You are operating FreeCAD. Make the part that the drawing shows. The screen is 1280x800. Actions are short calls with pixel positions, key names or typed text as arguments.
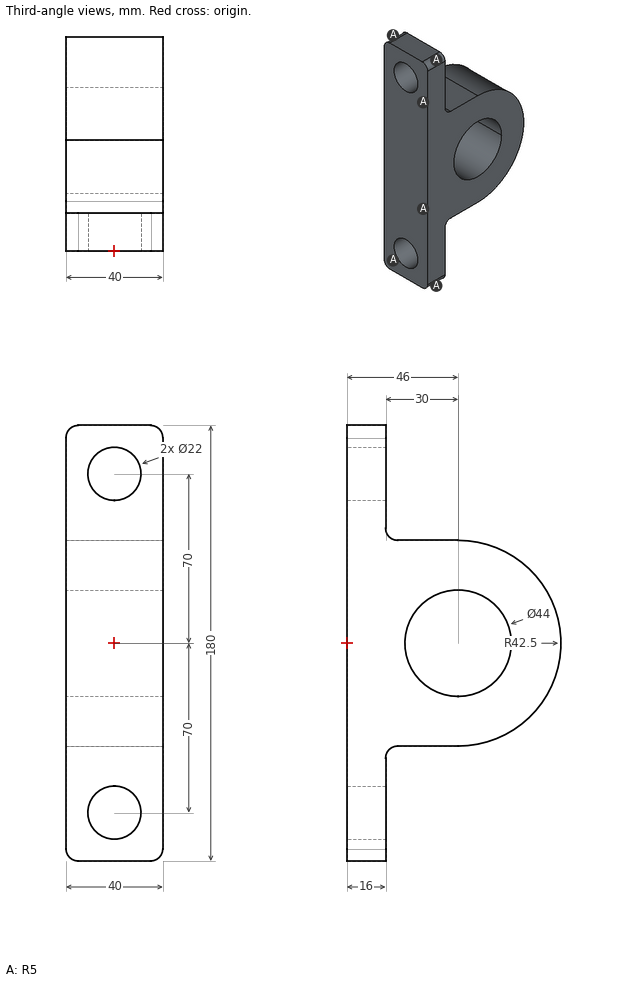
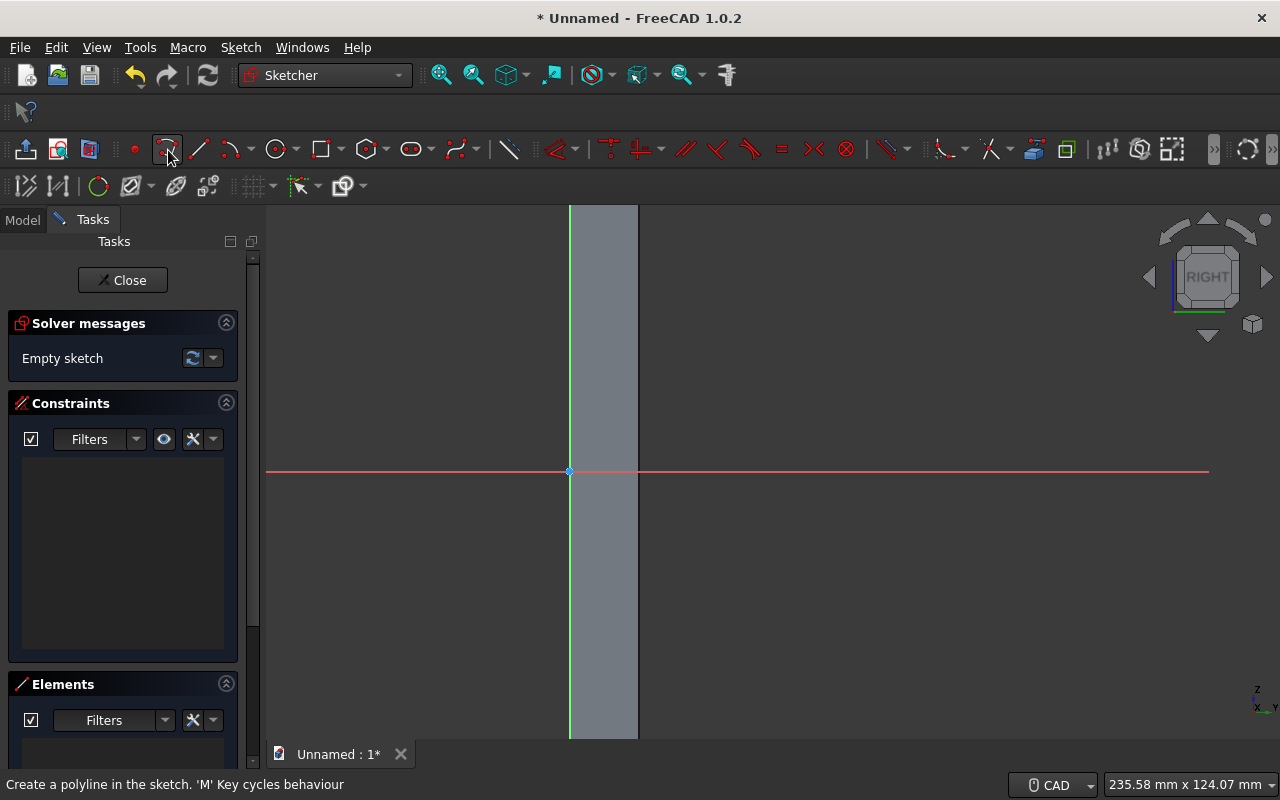
click(768, 289)
click(639, 289)
click(639, 655)
click(768, 655)
right_click(768, 655)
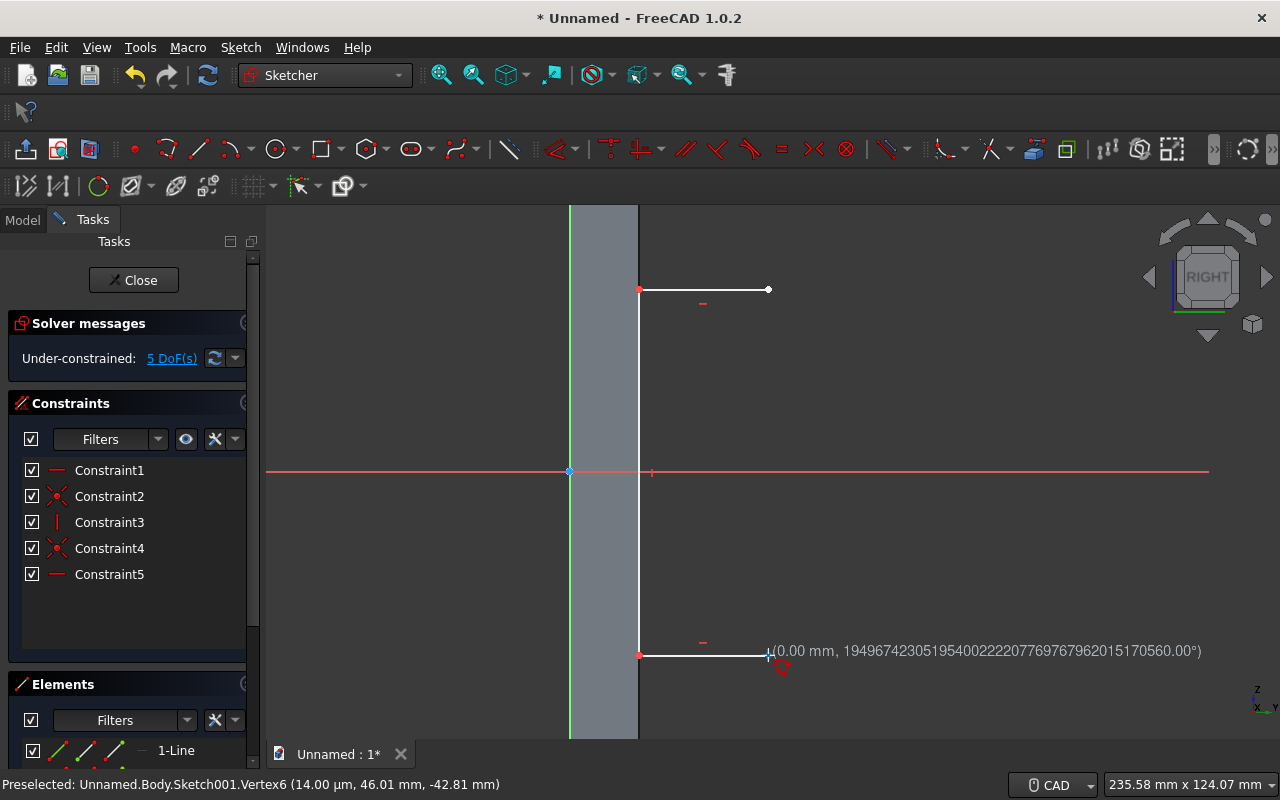
click(254, 150)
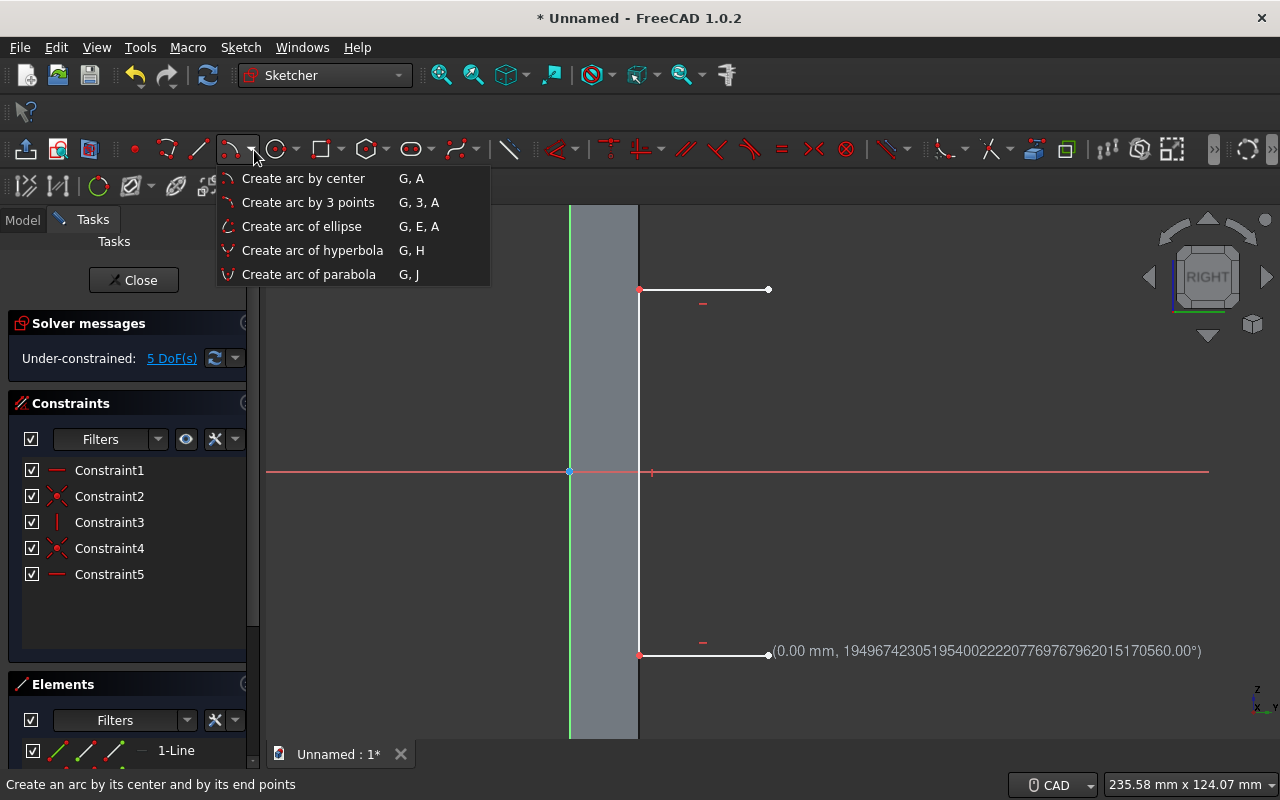
click(354, 202)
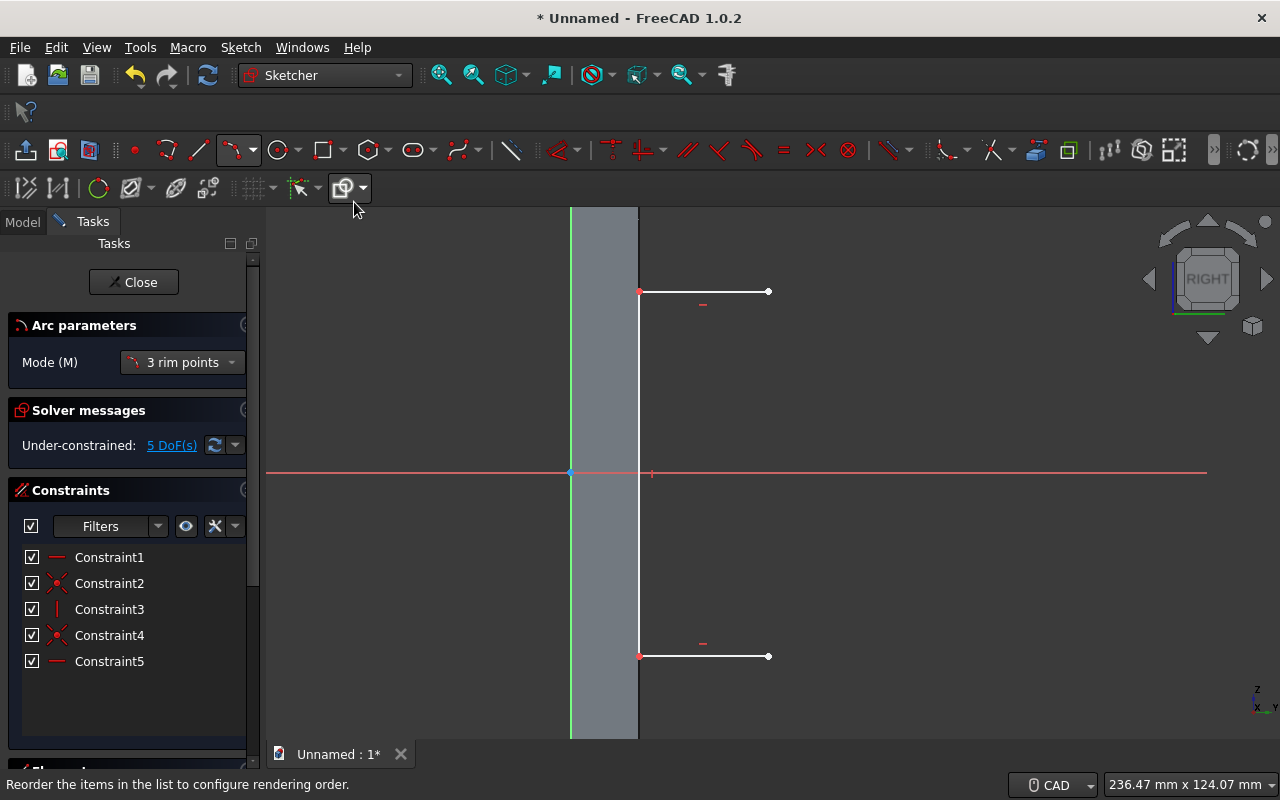
click(768, 656)
click(768, 292)
click(941, 529)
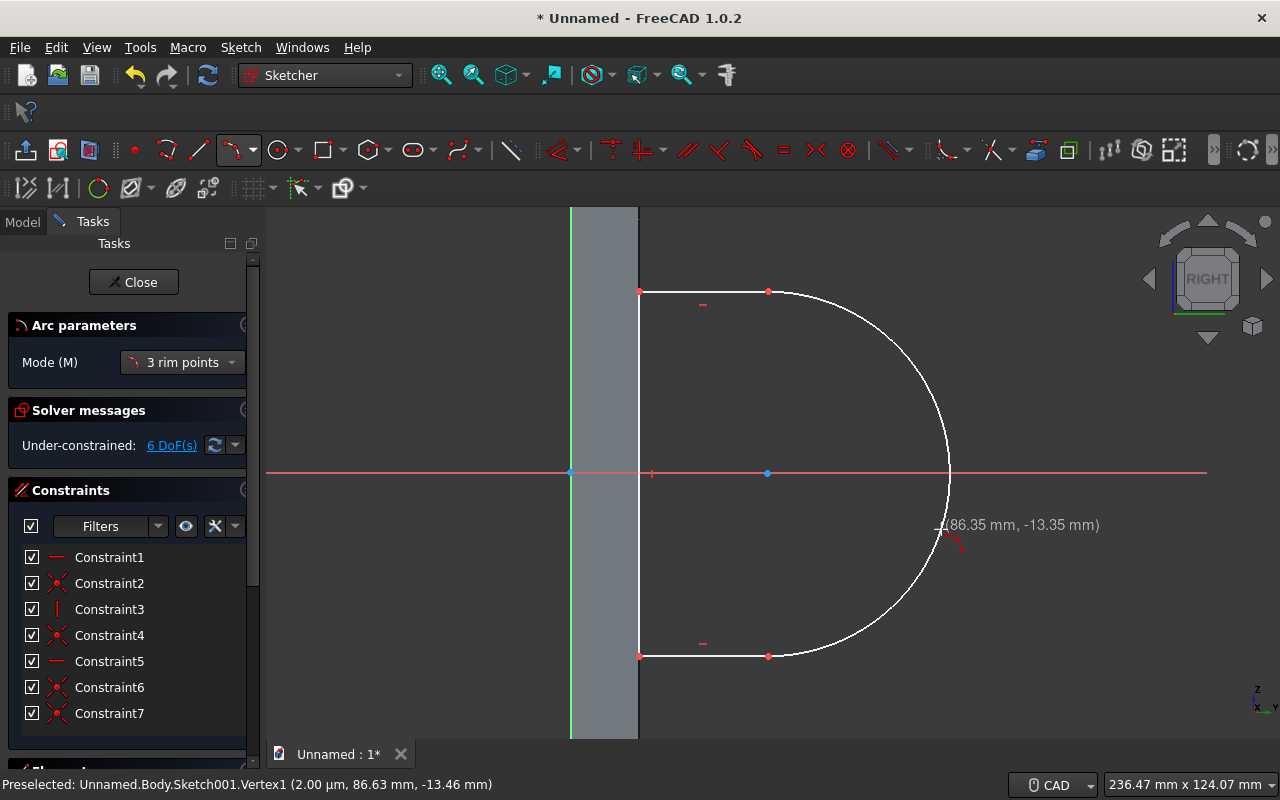
key(g)
key(c)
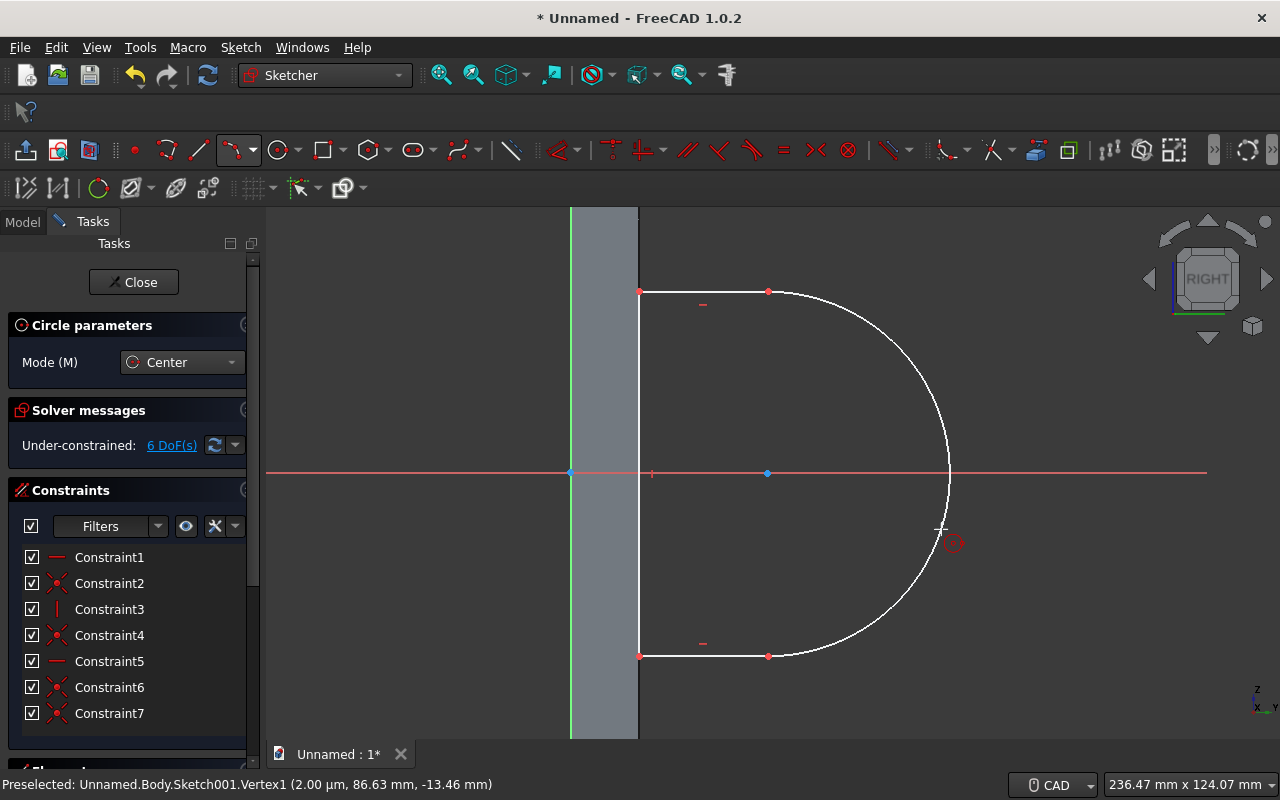
click(768, 473)
click(835, 406)
key(Escape)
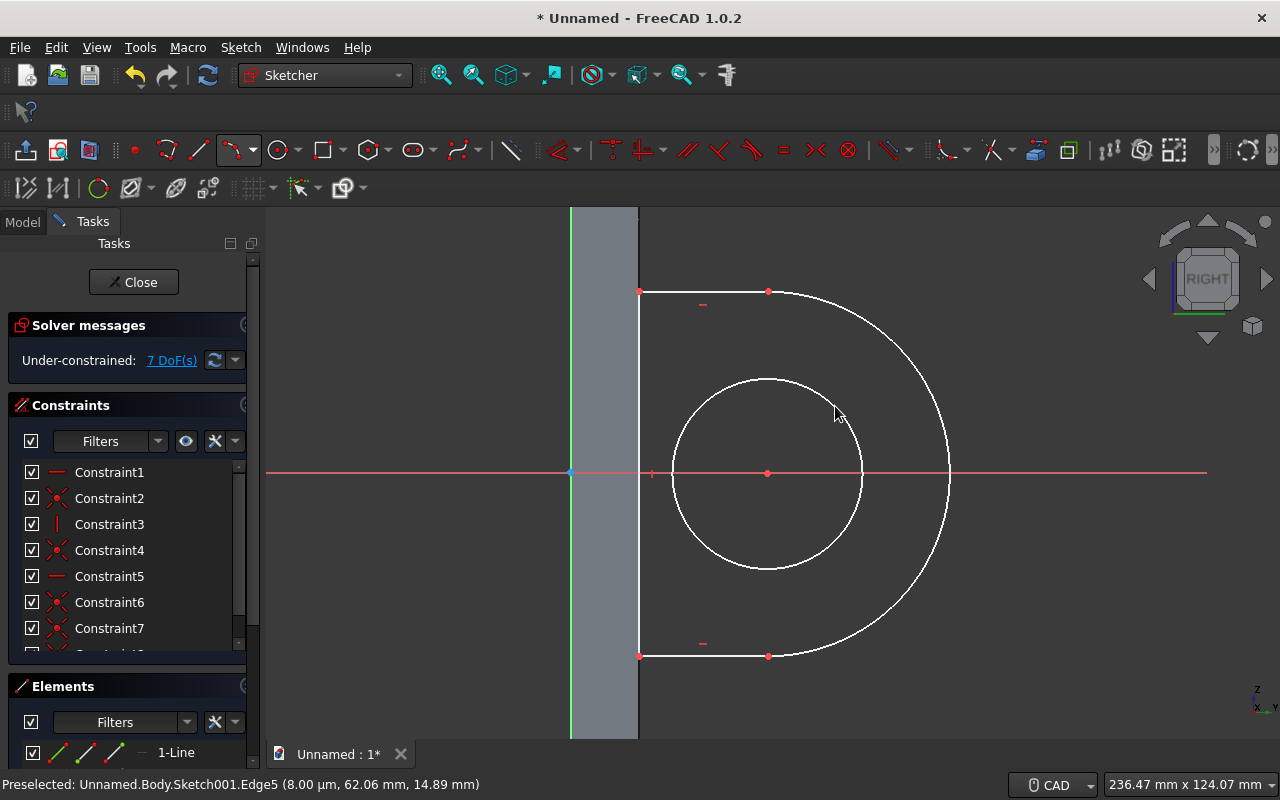
click(767, 474)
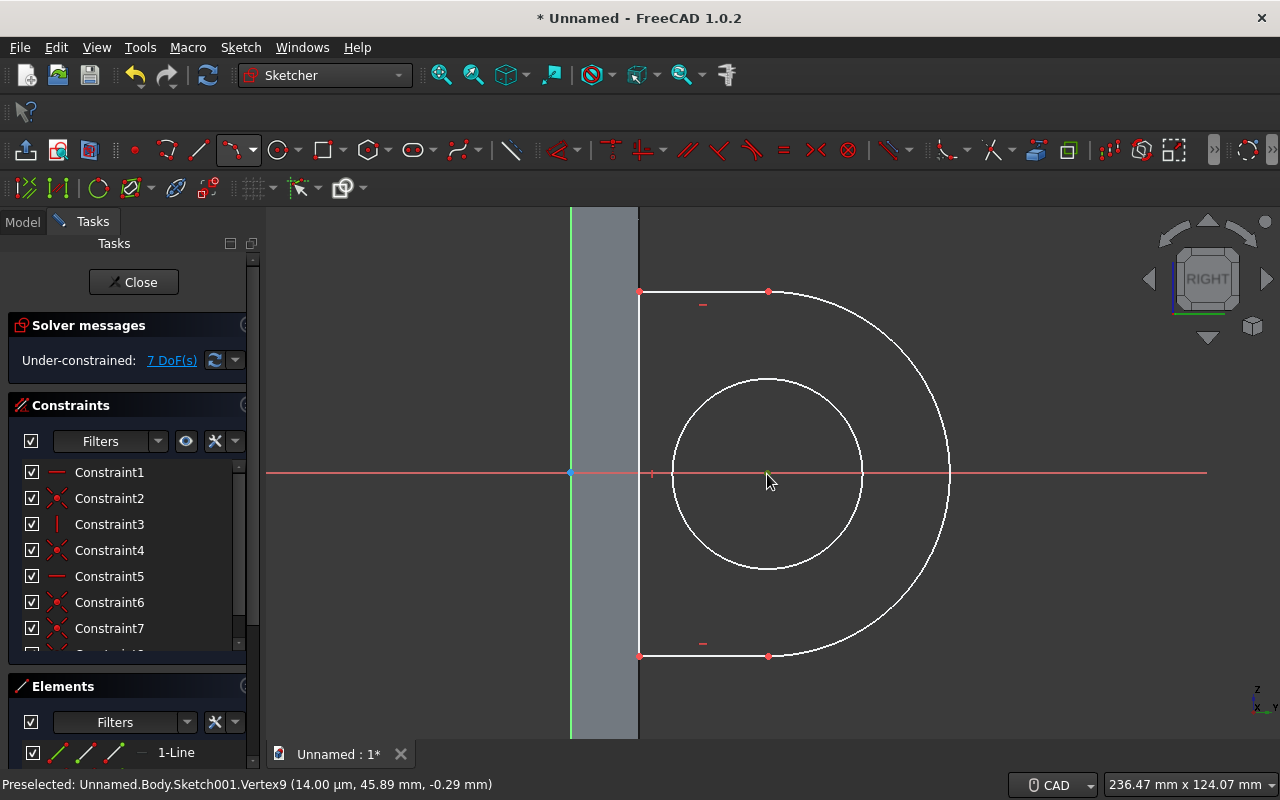
click(353, 473)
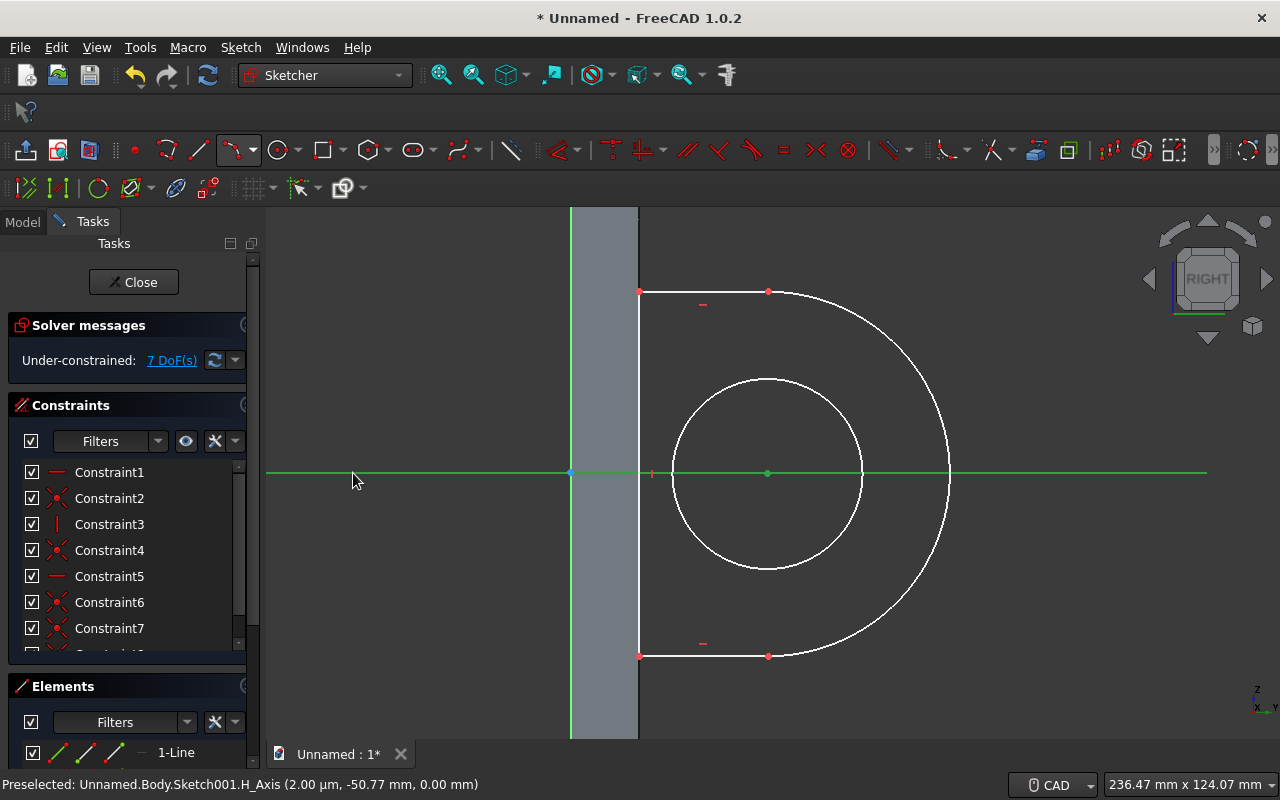
click(612, 150)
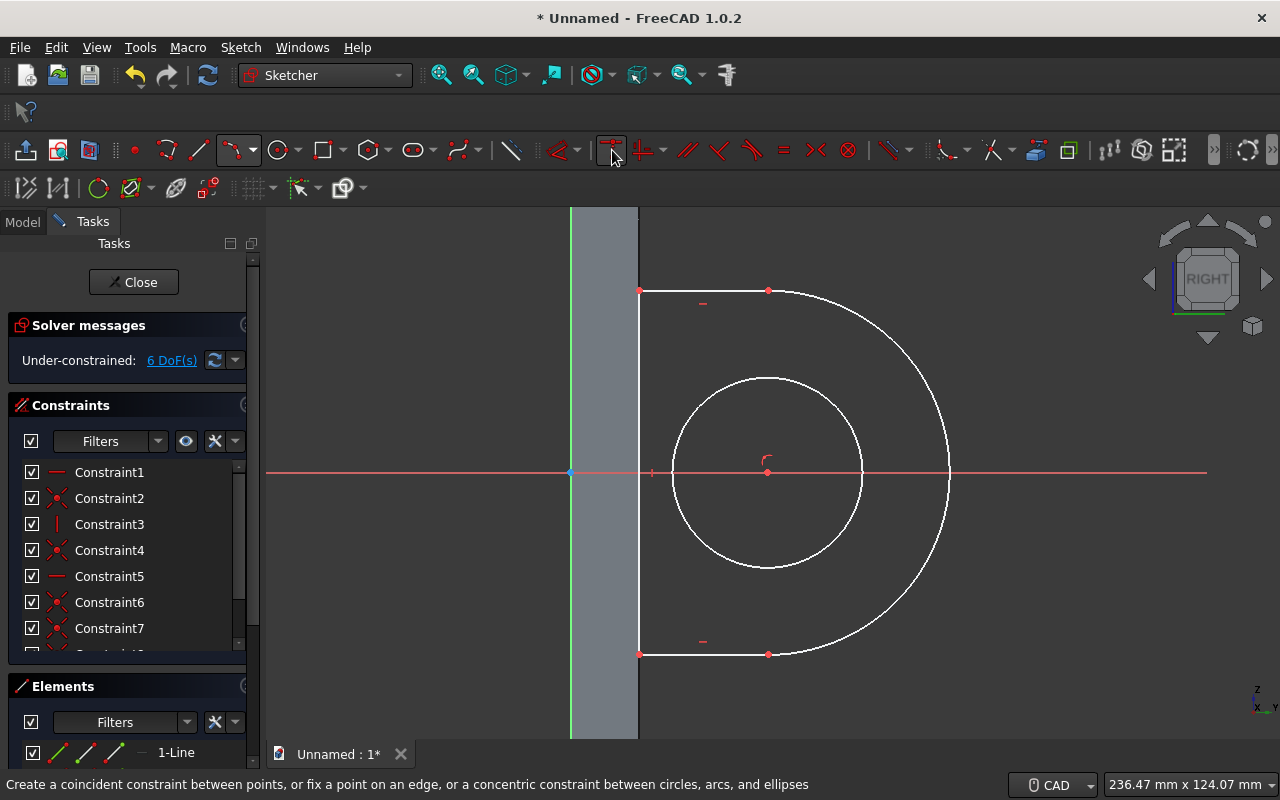
click(915, 580)